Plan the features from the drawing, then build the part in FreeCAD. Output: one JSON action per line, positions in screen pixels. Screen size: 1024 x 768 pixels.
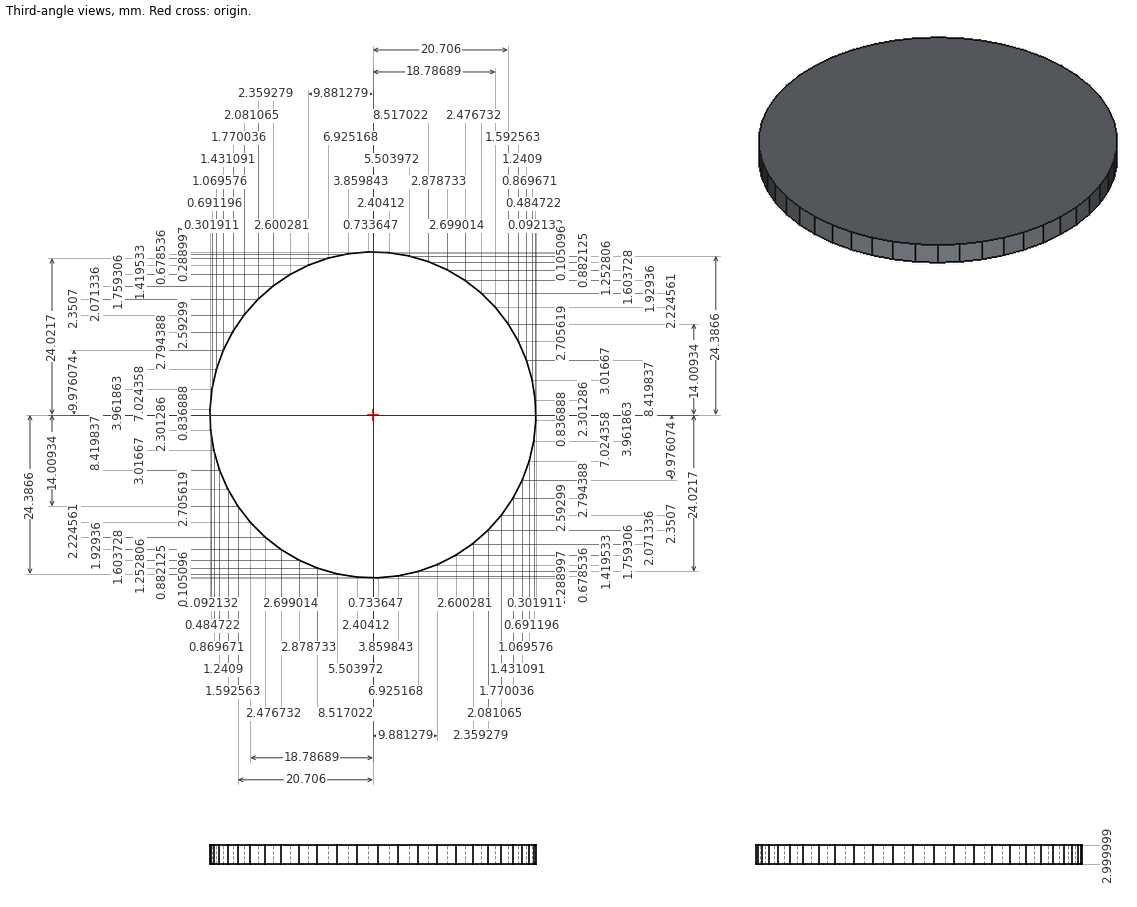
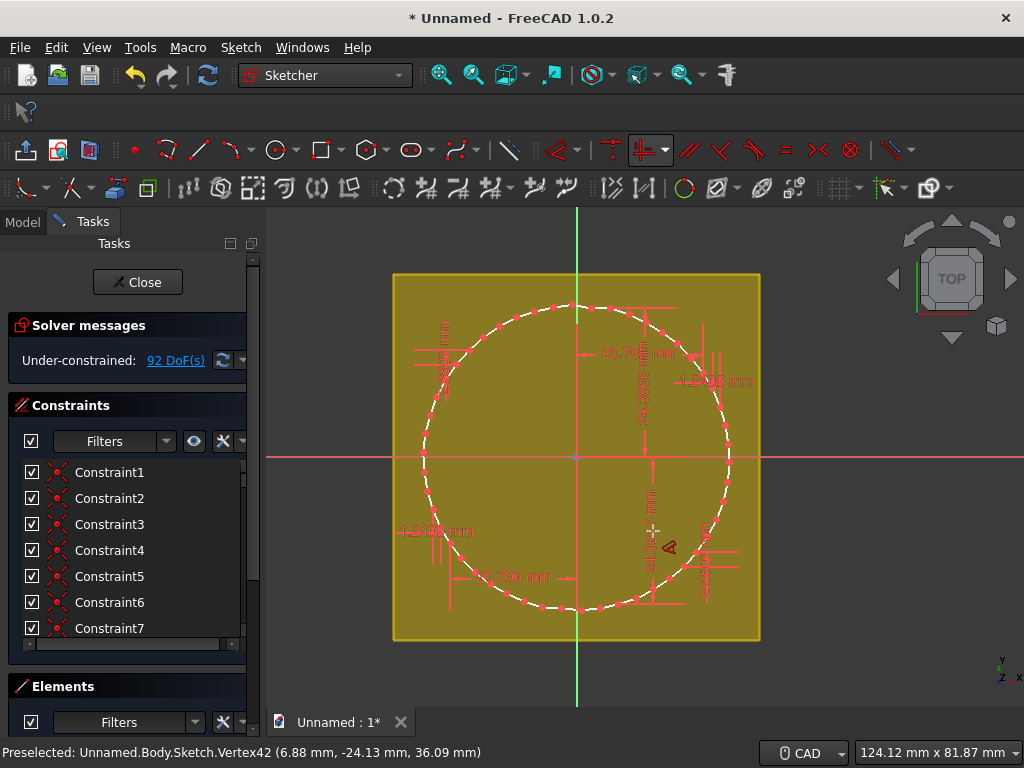
{"action": "scroll", "coordinate": [562, 609], "scroll_direction": "up", "scroll_amount": 5}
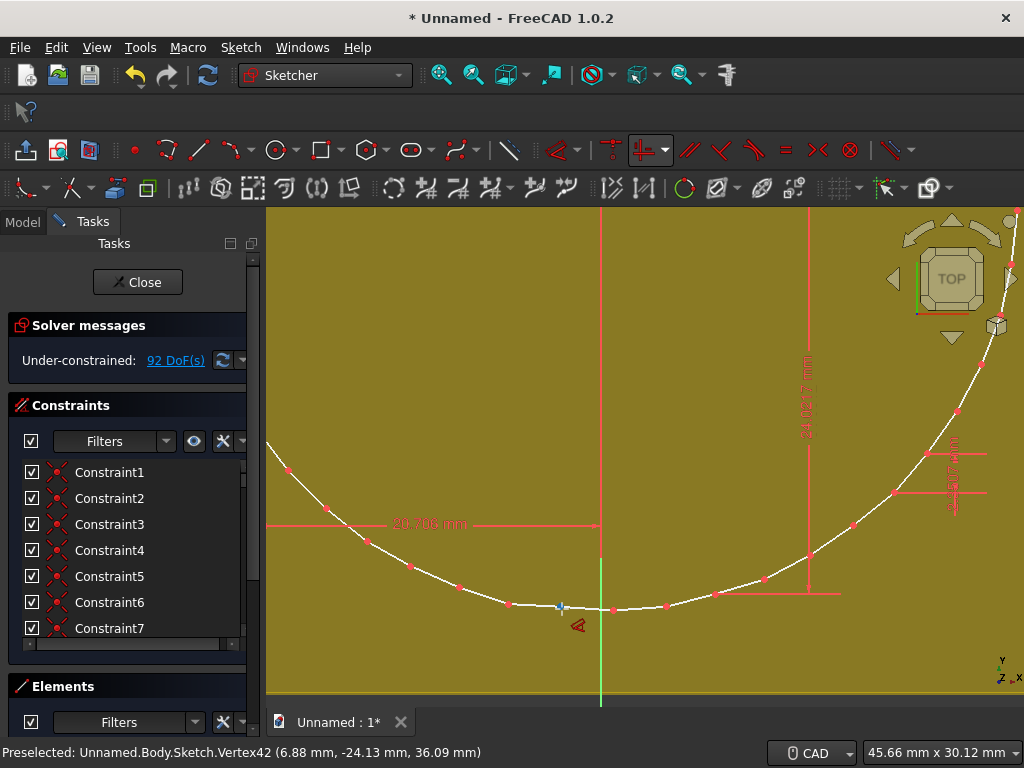
{"action": "left_click", "coordinate": [560, 607]}
{"action": "left_click", "coordinate": [581, 641]}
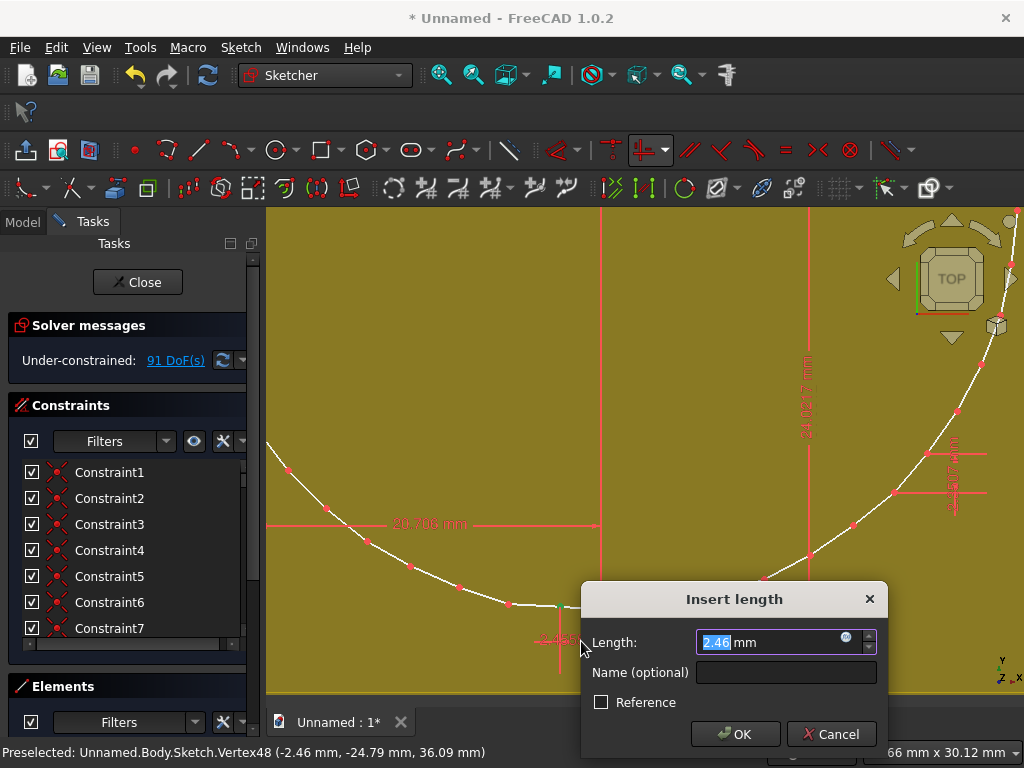
{"action": "type", "text": "2.40412"}
{"action": "key", "text": "Return"}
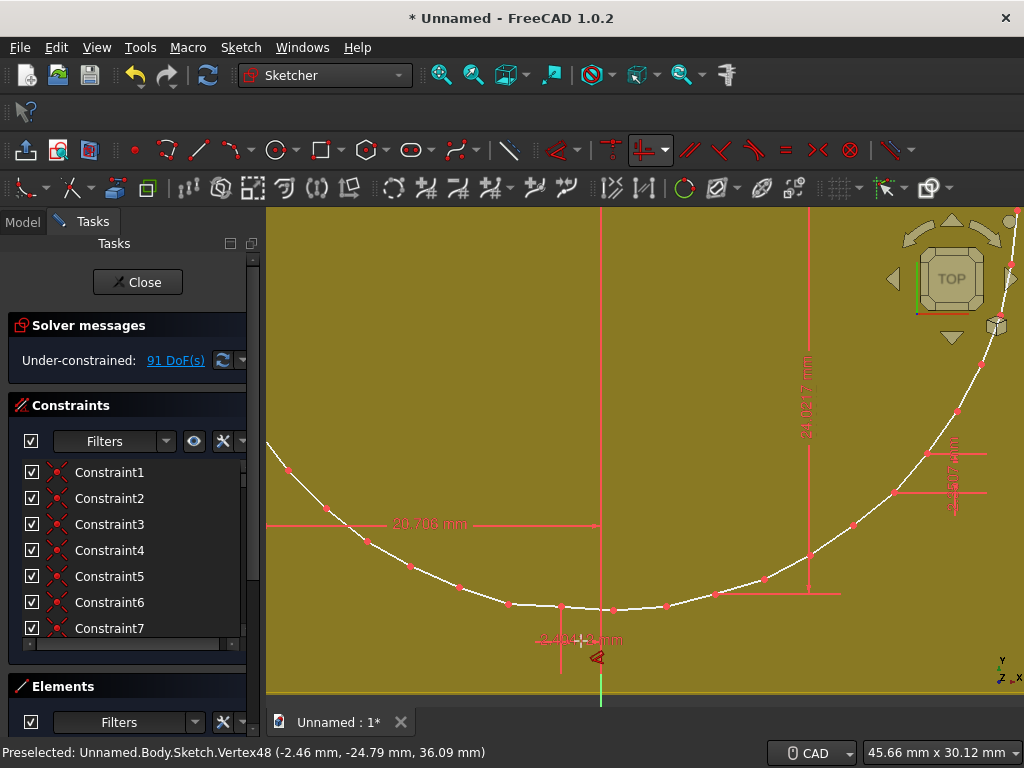
{"action": "left_click", "coordinate": [509, 604]}
{"action": "left_click", "coordinate": [475, 420]}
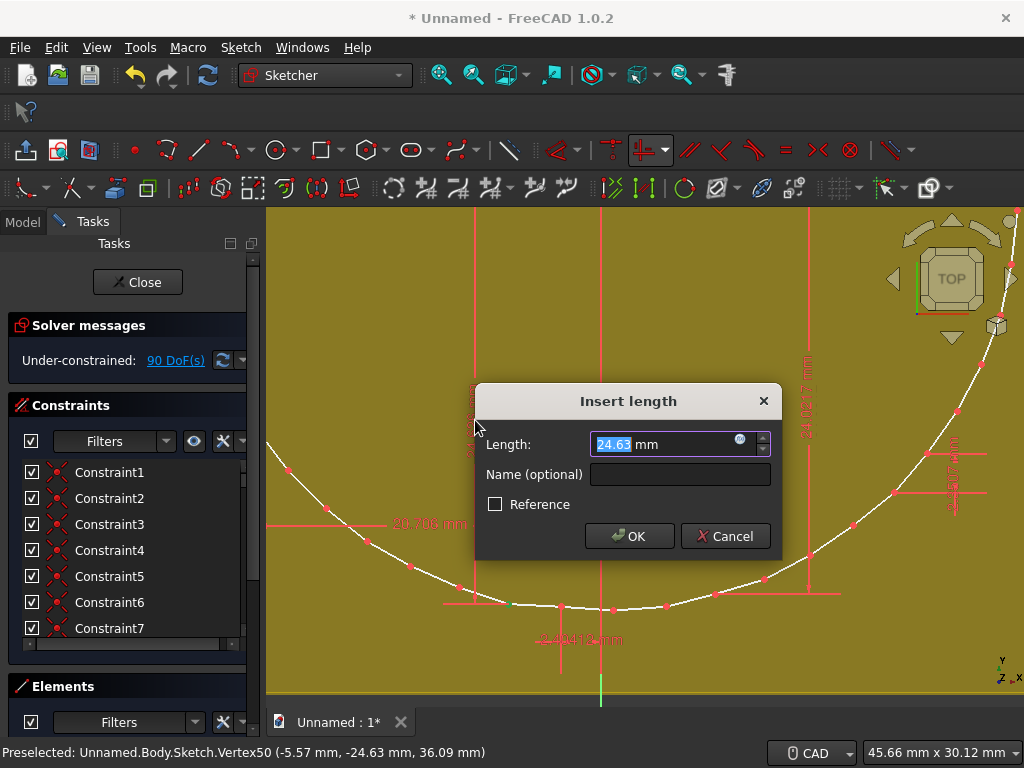
{"action": "type", "text": "24.3866"}
{"action": "key", "text": "Return"}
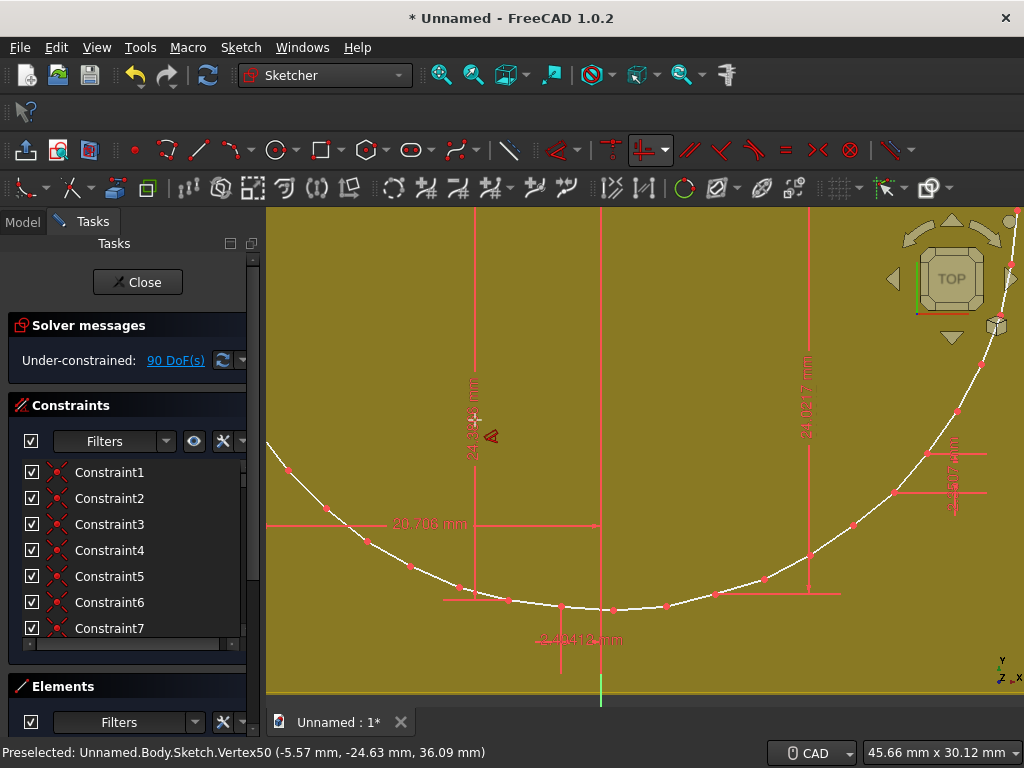
{"action": "scroll", "coordinate": [562, 609], "scroll_direction": "down", "scroll_amount": 5}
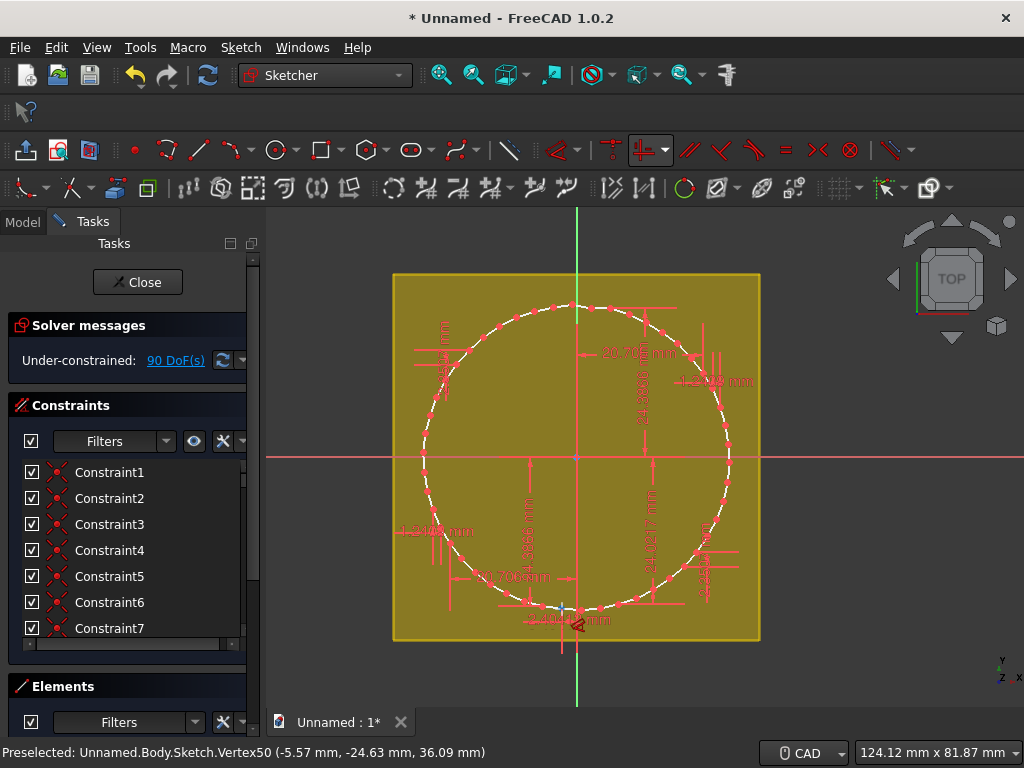
{"action": "left_click", "coordinate": [534, 312]}
{"action": "left_click", "coordinate": [500, 385]}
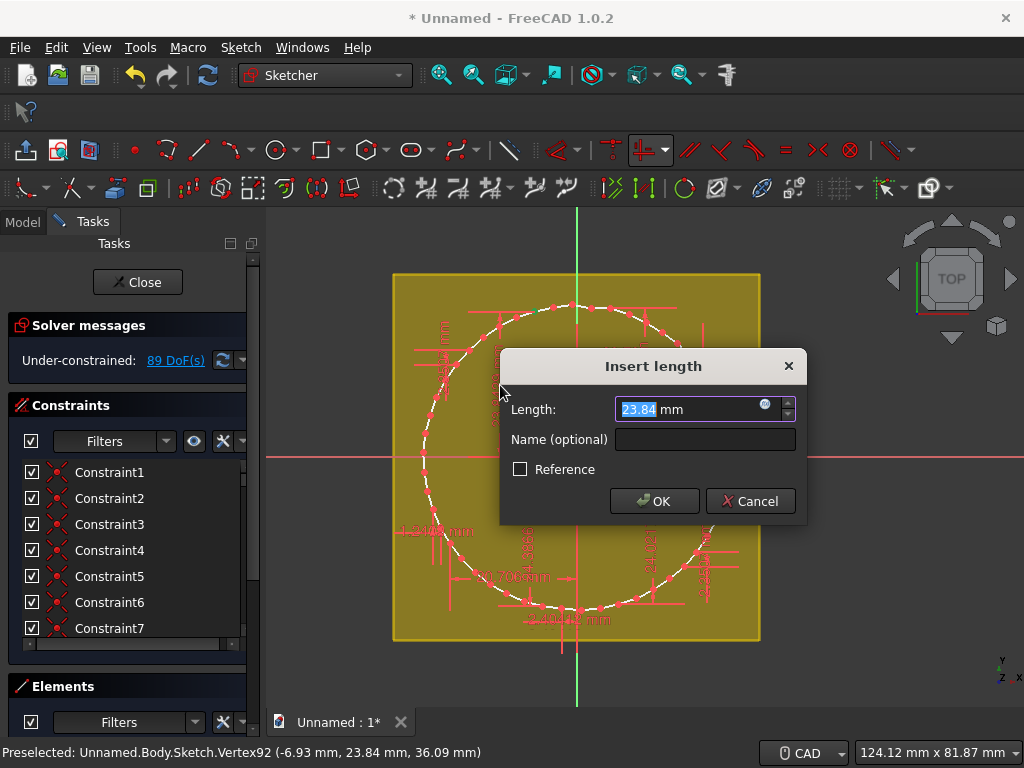
{"action": "type", "text": "24.0217"}
{"action": "key", "text": "Return"}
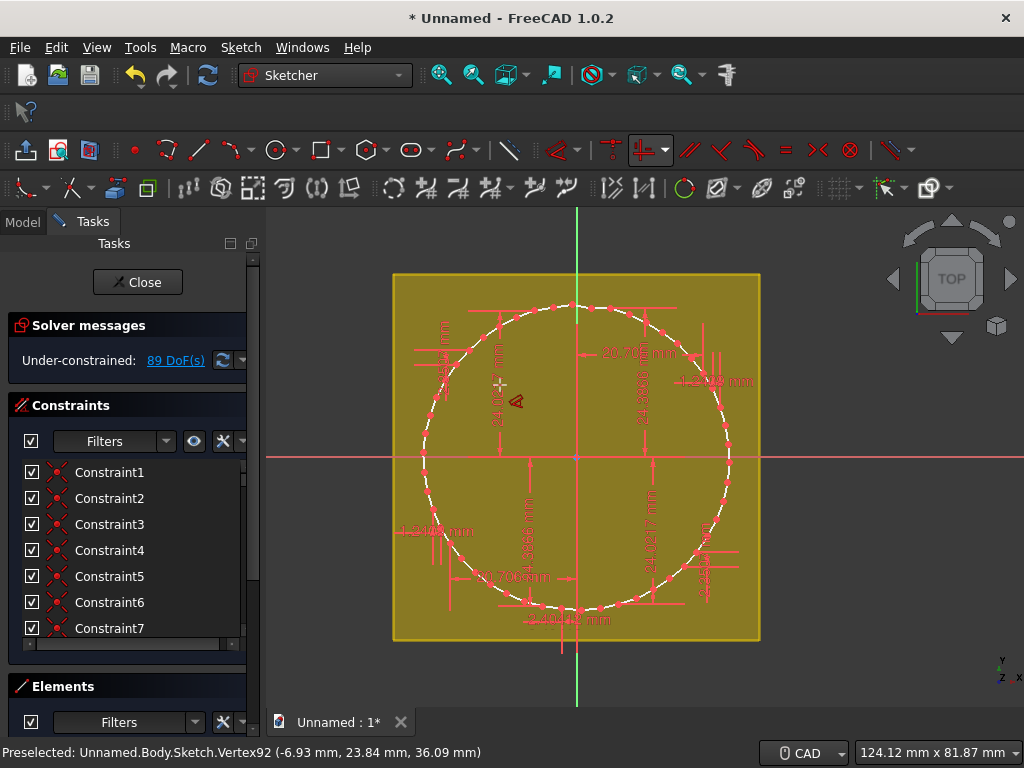
{"action": "scroll", "coordinate": [592, 308], "scroll_direction": "up", "scroll_amount": 5}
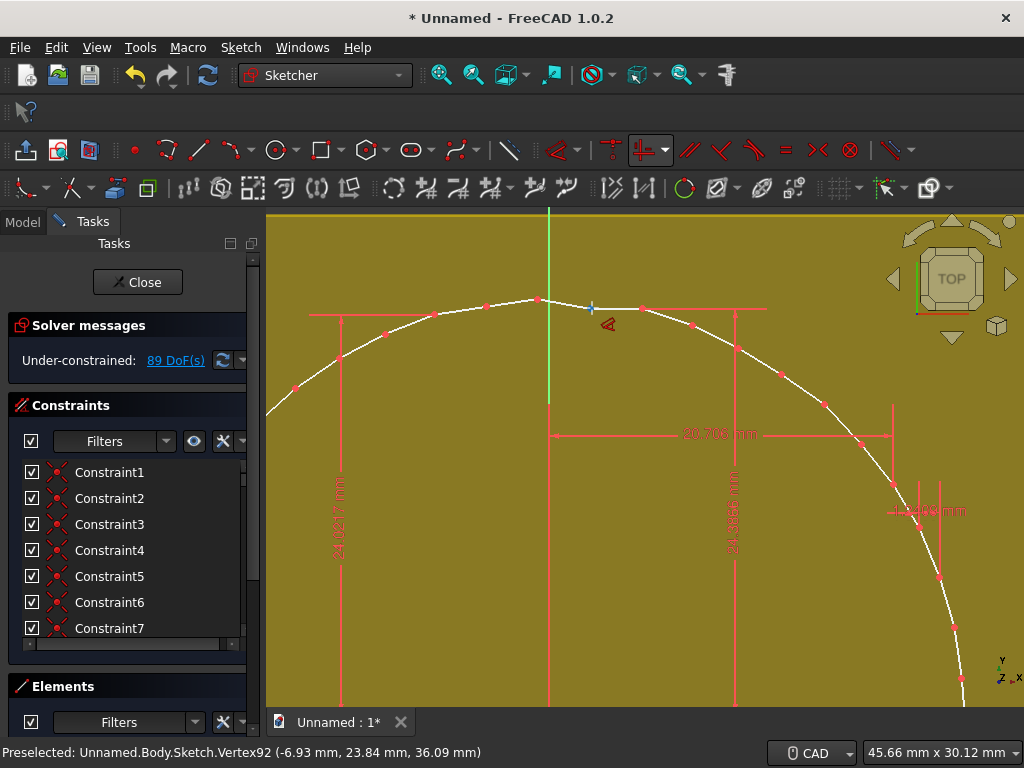
{"action": "left_click", "coordinate": [590, 309]}
{"action": "left_click", "coordinate": [570, 275]}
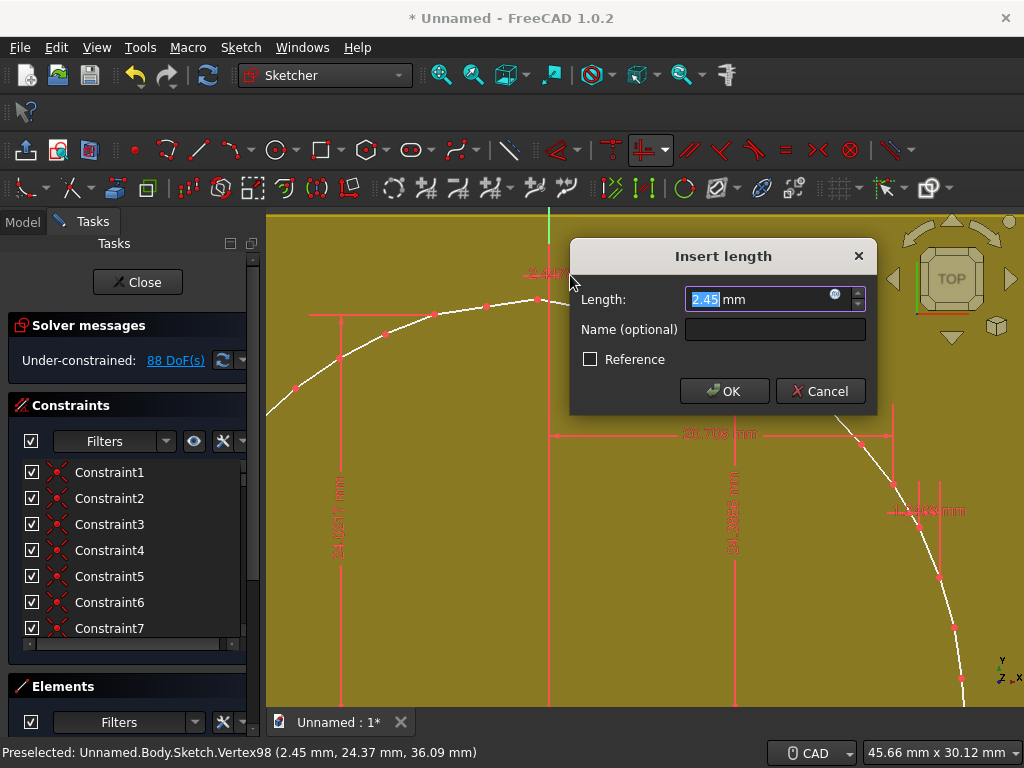
{"action": "type", "text": "2.40412"}
{"action": "key", "text": "Return"}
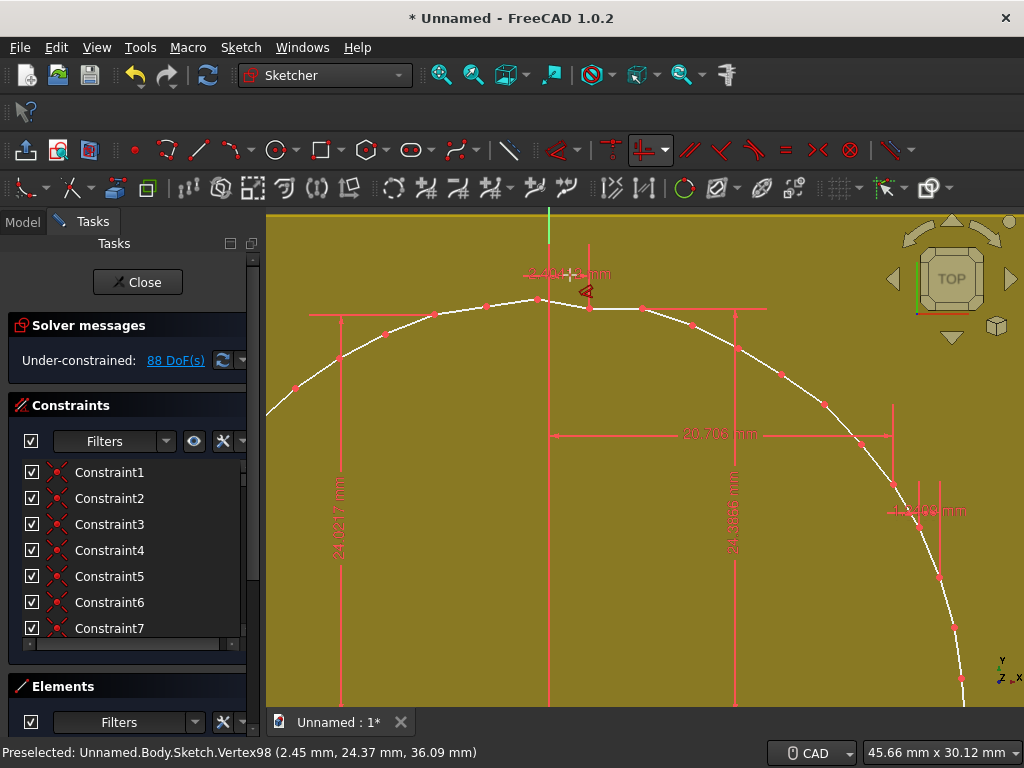
{"action": "scroll", "coordinate": [795, 384], "scroll_direction": "up", "scroll_amount": 2}